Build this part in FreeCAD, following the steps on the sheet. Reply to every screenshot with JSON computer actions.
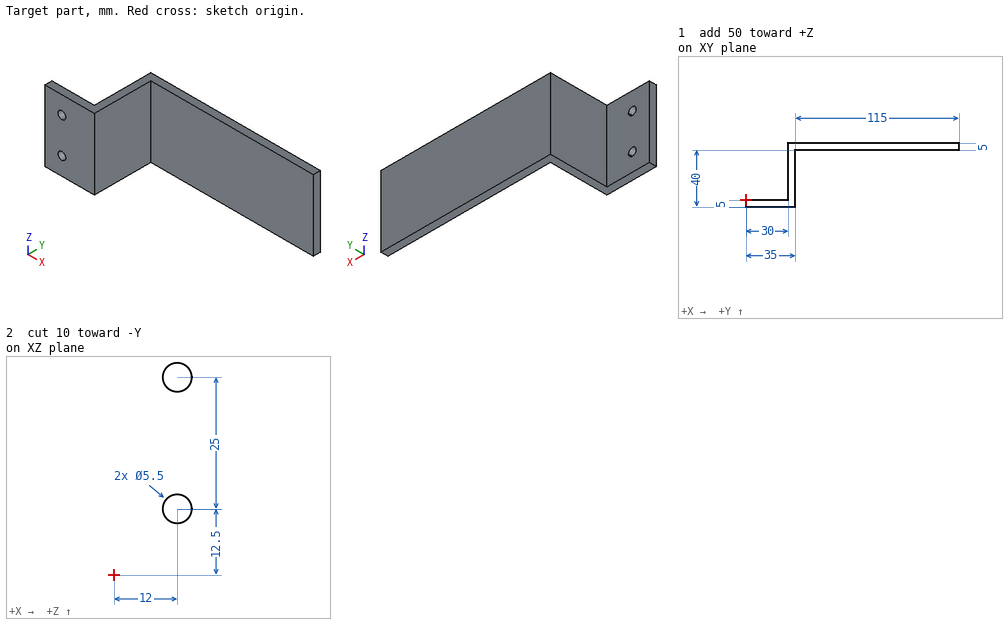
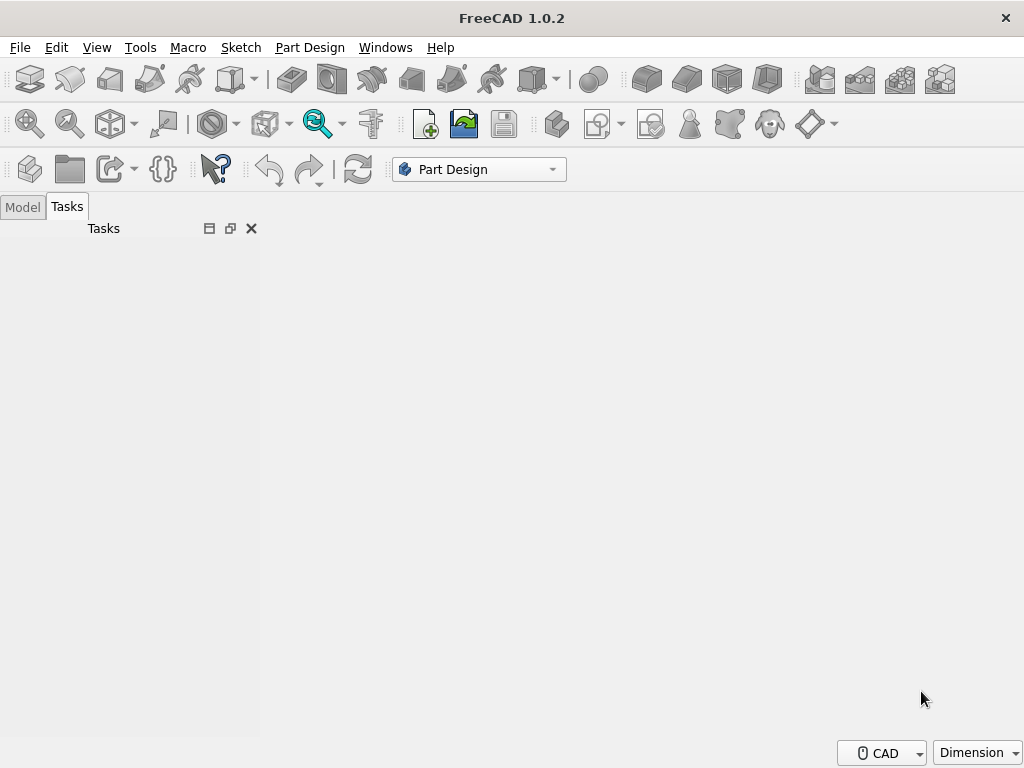
{"action": "left_click", "coordinate": [424, 124]}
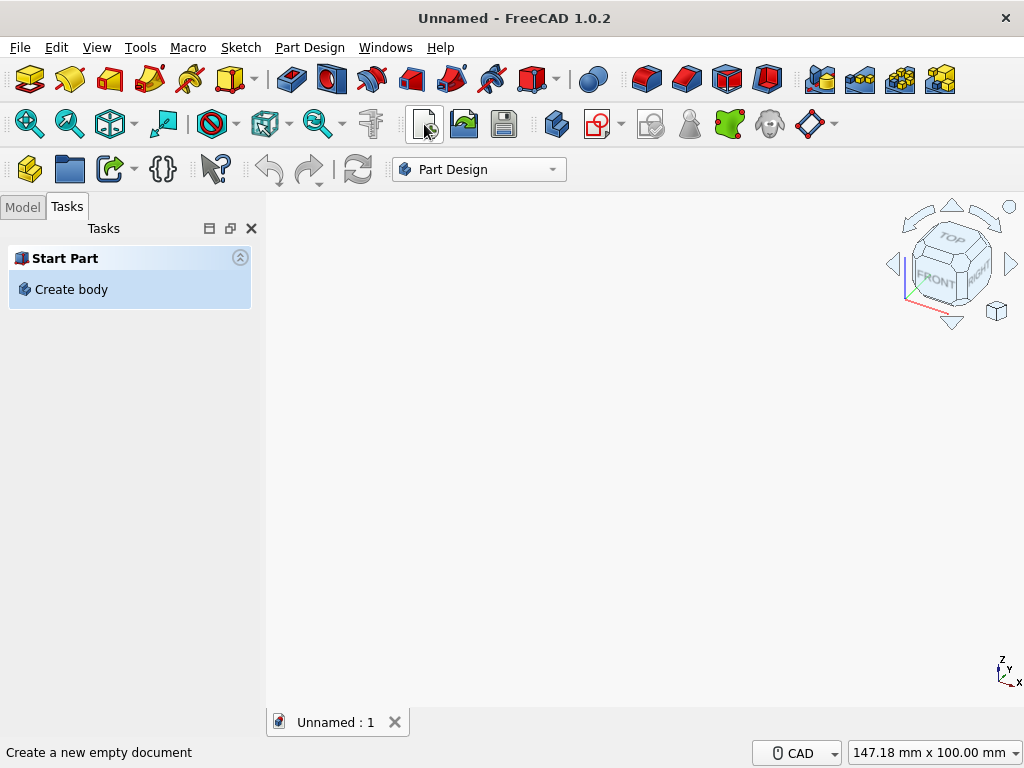
{"action": "left_click", "coordinate": [598, 124]}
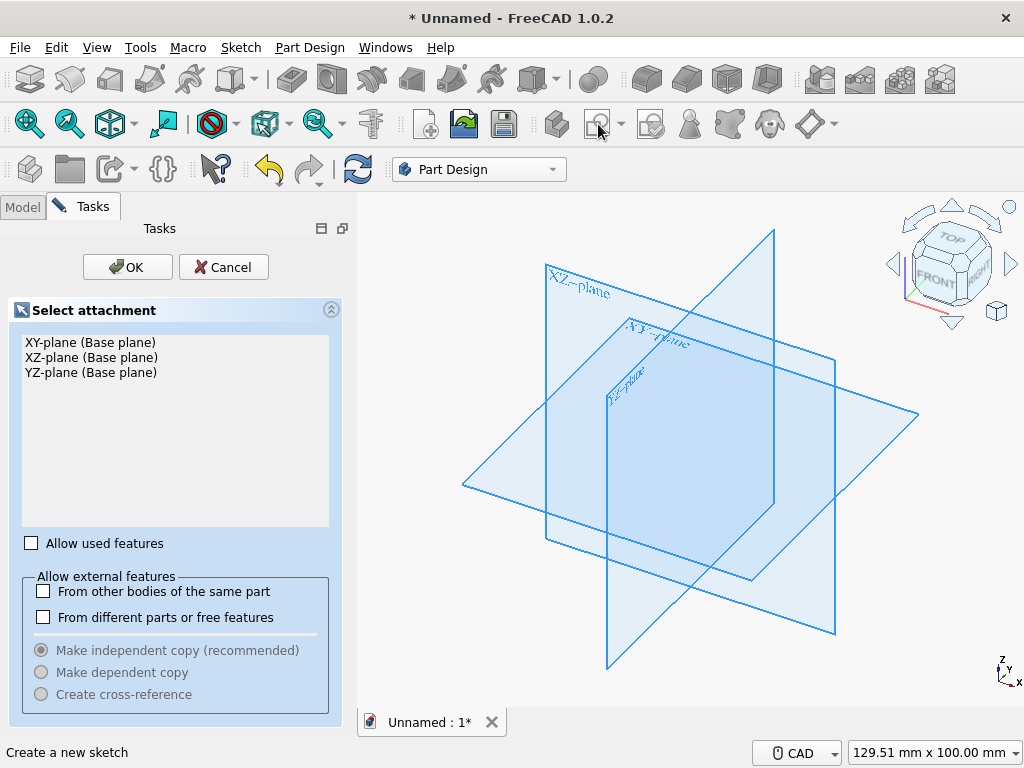
{"action": "left_click", "coordinate": [82, 342]}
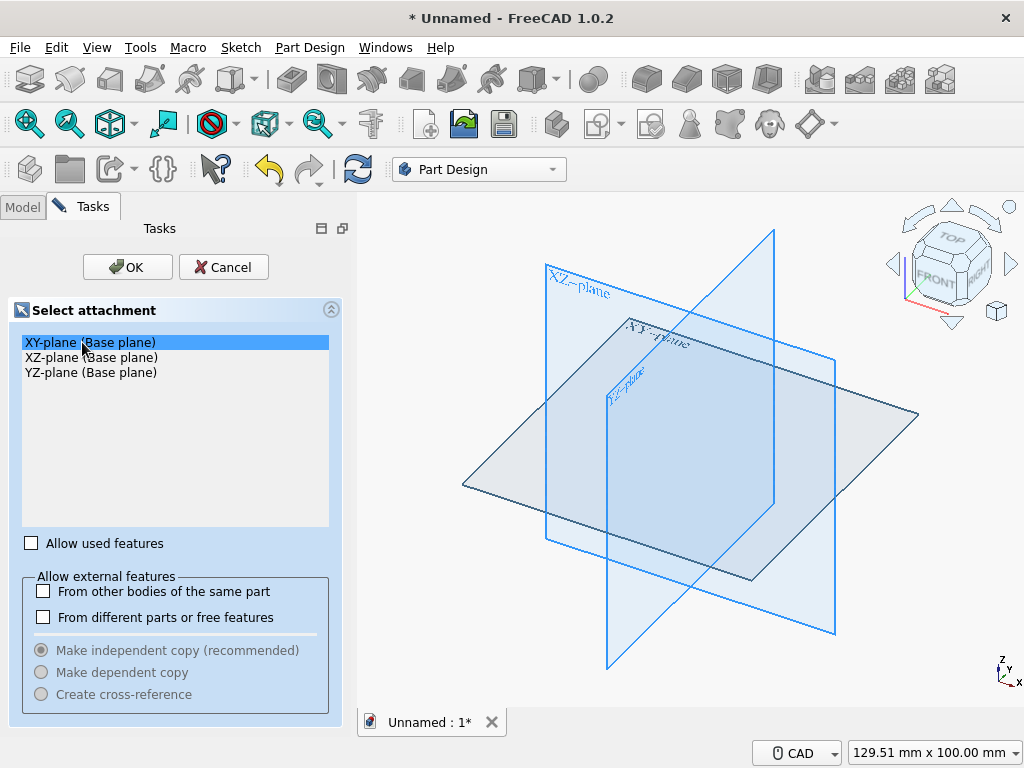
{"action": "left_click", "coordinate": [128, 267]}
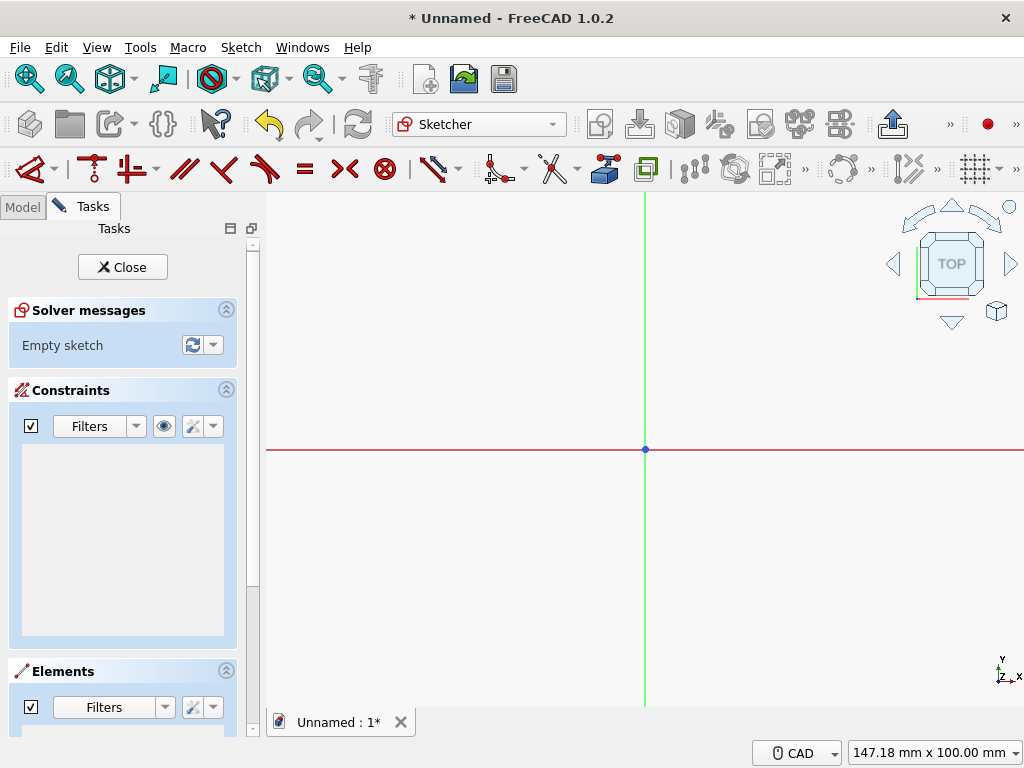
{"action": "scroll", "coordinate": [294, 523], "scroll_direction": "down", "scroll_amount": 4}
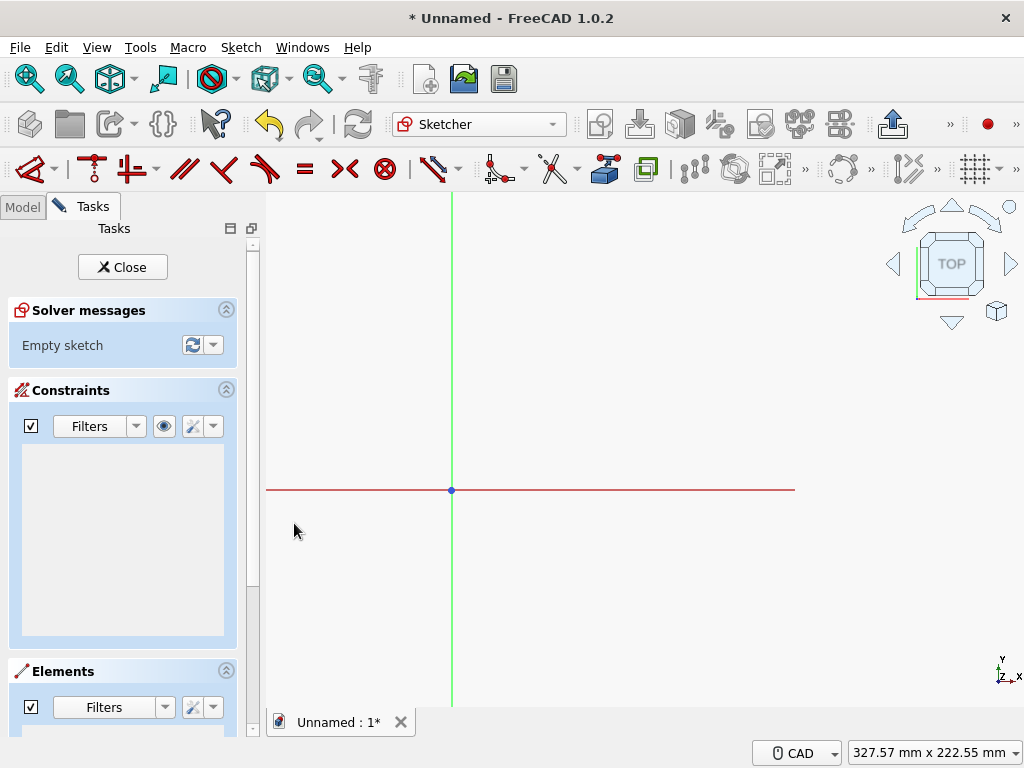
{"action": "key", "text": "g m"}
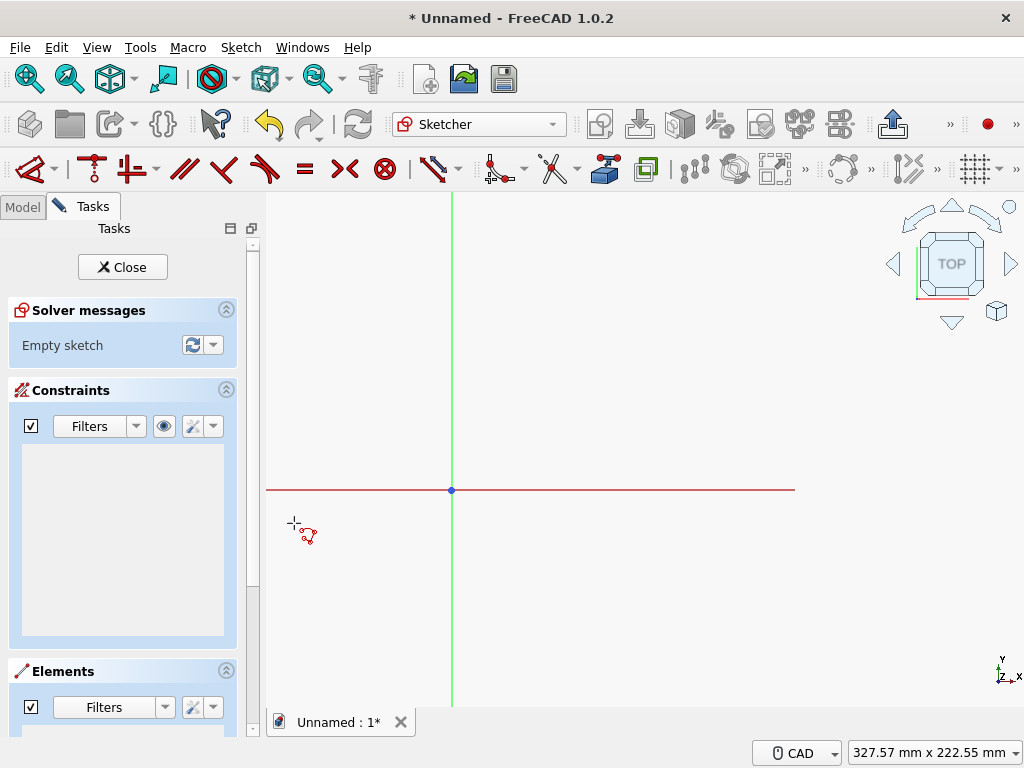
{"action": "left_click", "coordinate": [452, 490]}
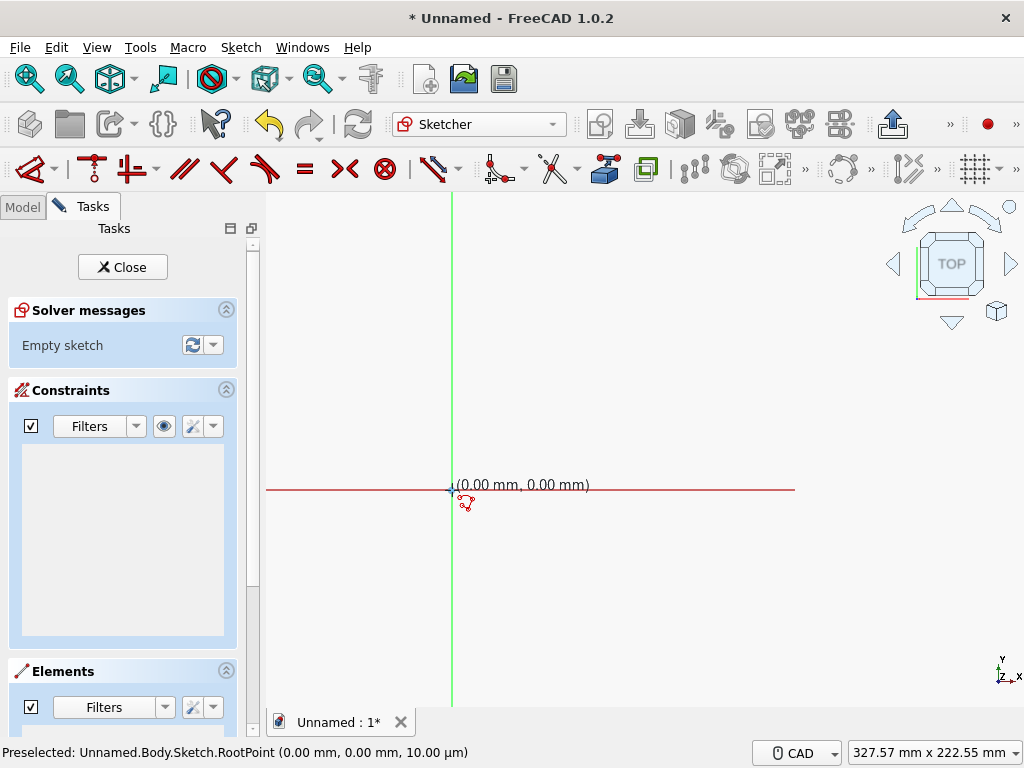
{"action": "scroll", "coordinate": [452, 502], "scroll_direction": "up", "scroll_amount": 2}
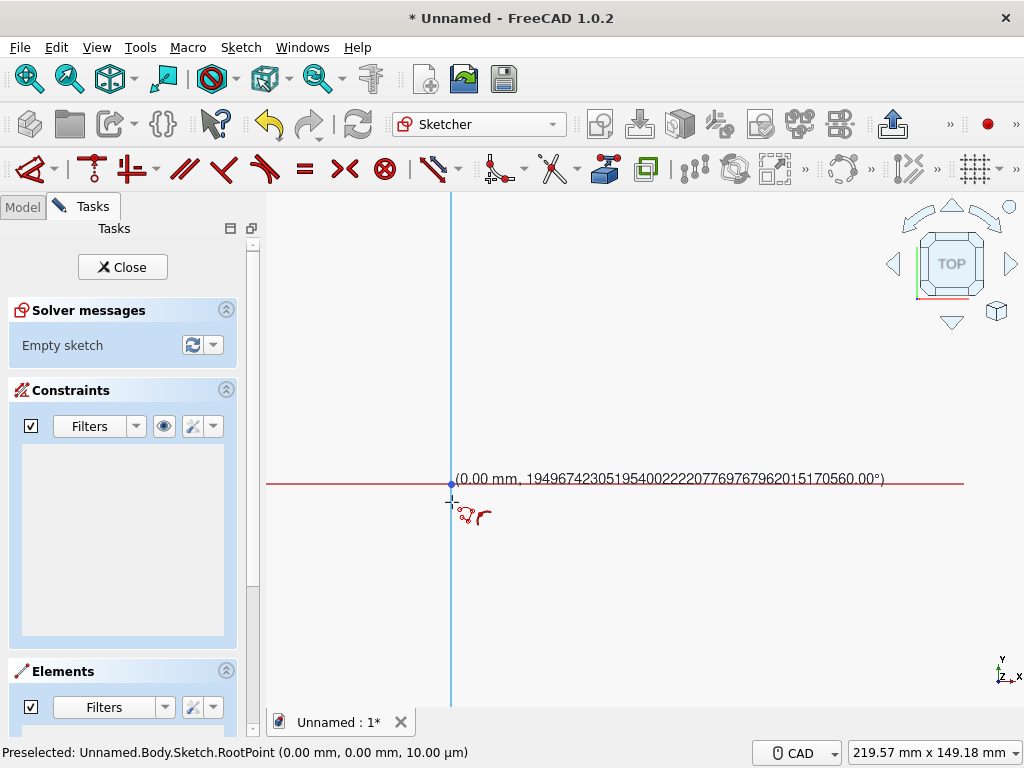
{"action": "left_click", "coordinate": [460, 502]}
{"action": "left_click", "coordinate": [572, 502]}
{"action": "left_click", "coordinate": [572, 363]}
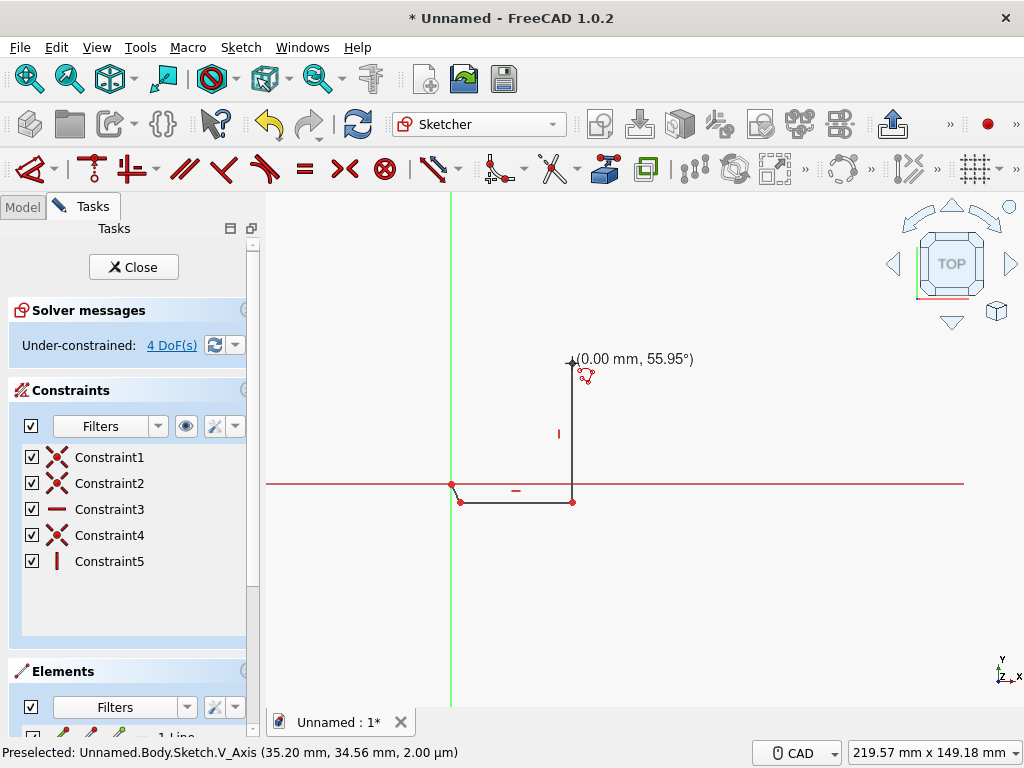
{"action": "scroll", "coordinate": [304, 502], "scroll_direction": "down", "scroll_amount": 2}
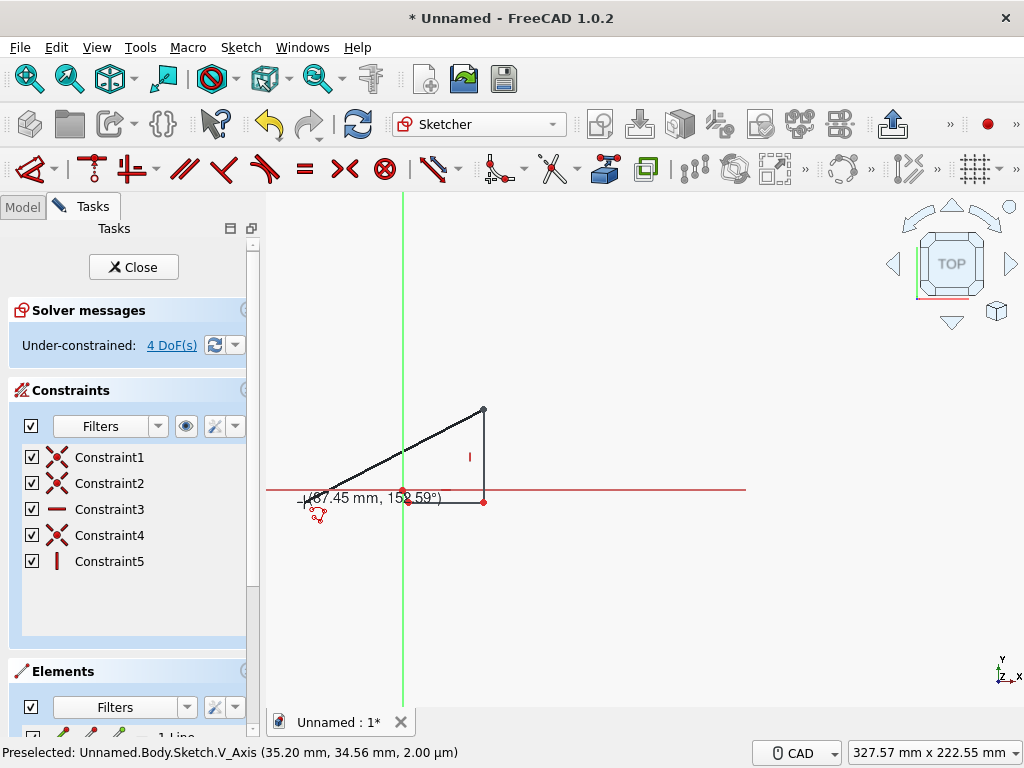
{"action": "left_click", "coordinate": [750, 409]}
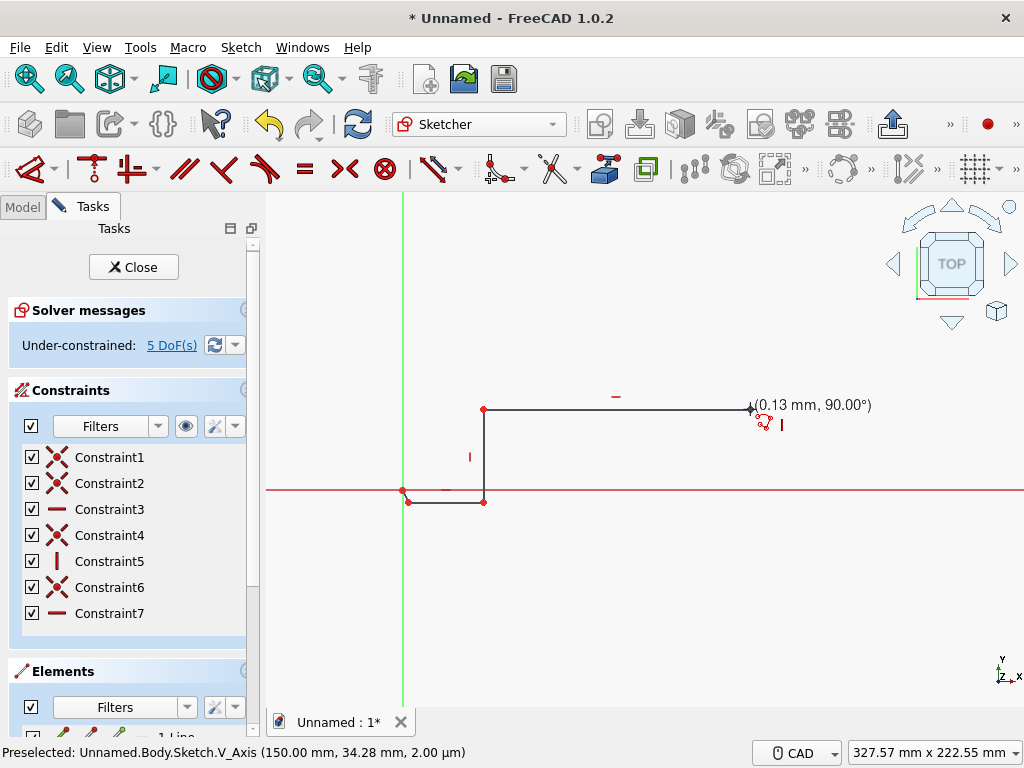
{"action": "scroll", "coordinate": [750, 398], "scroll_direction": "up", "scroll_amount": 2}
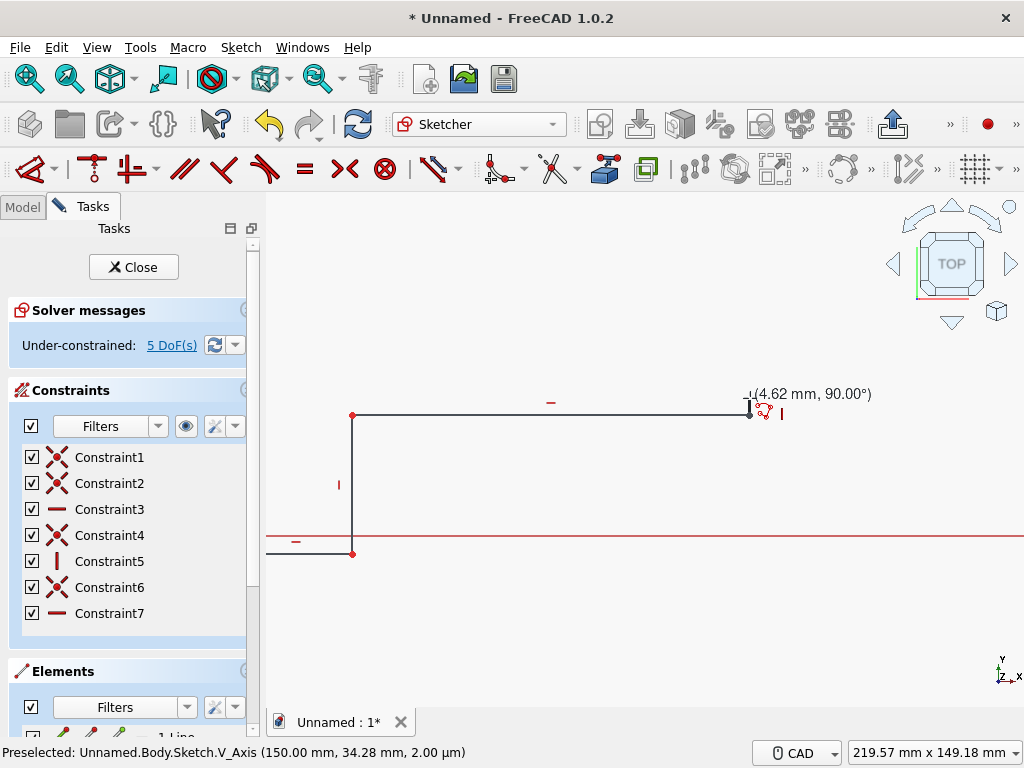
{"action": "left_click", "coordinate": [750, 397]}
{"action": "left_click", "coordinate": [335, 397]}
{"action": "left_click", "coordinate": [335, 527]}